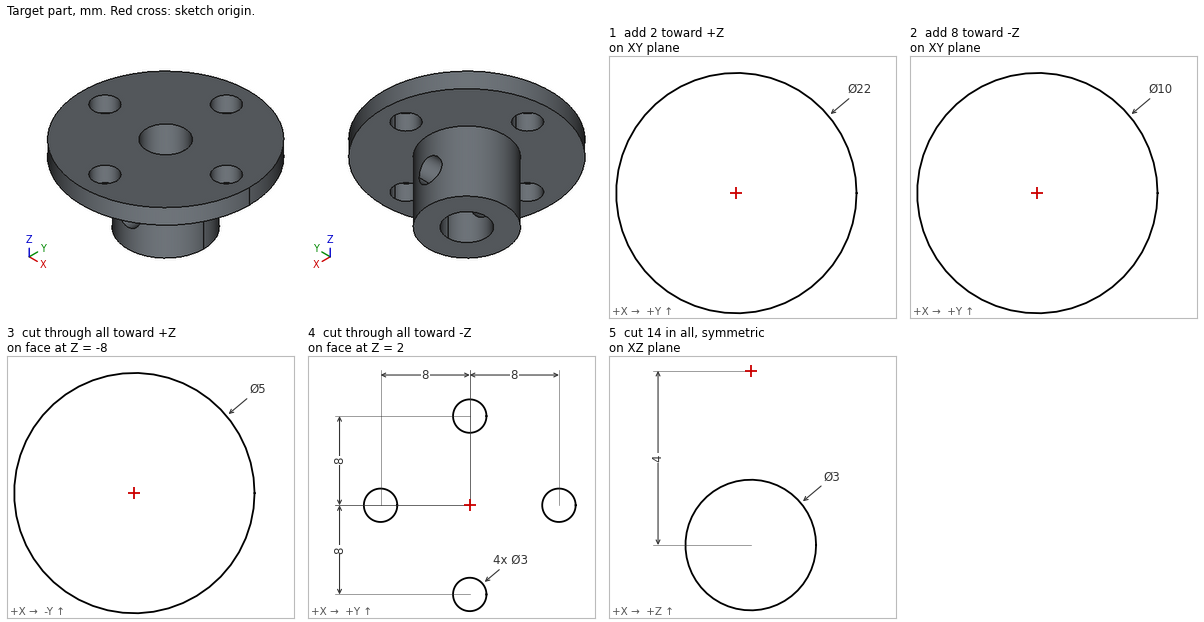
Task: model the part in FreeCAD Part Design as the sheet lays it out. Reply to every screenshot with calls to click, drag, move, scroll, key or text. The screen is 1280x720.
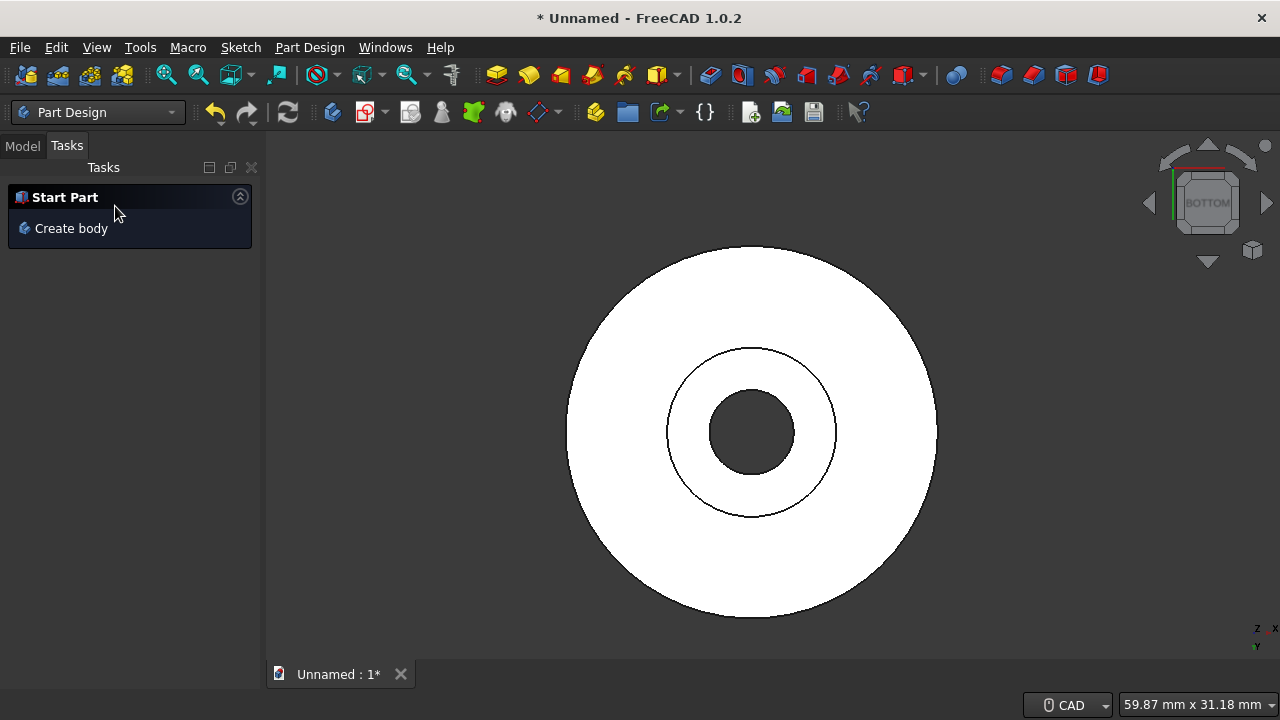
key(0)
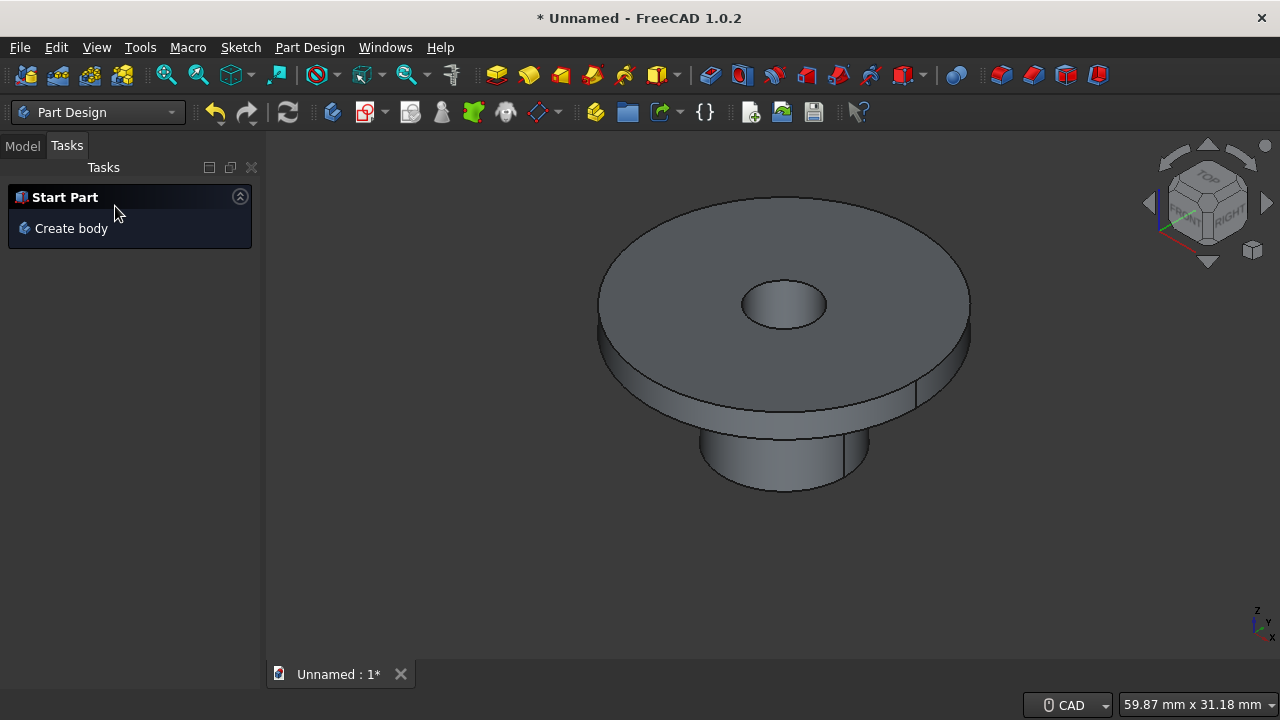
click(897, 282)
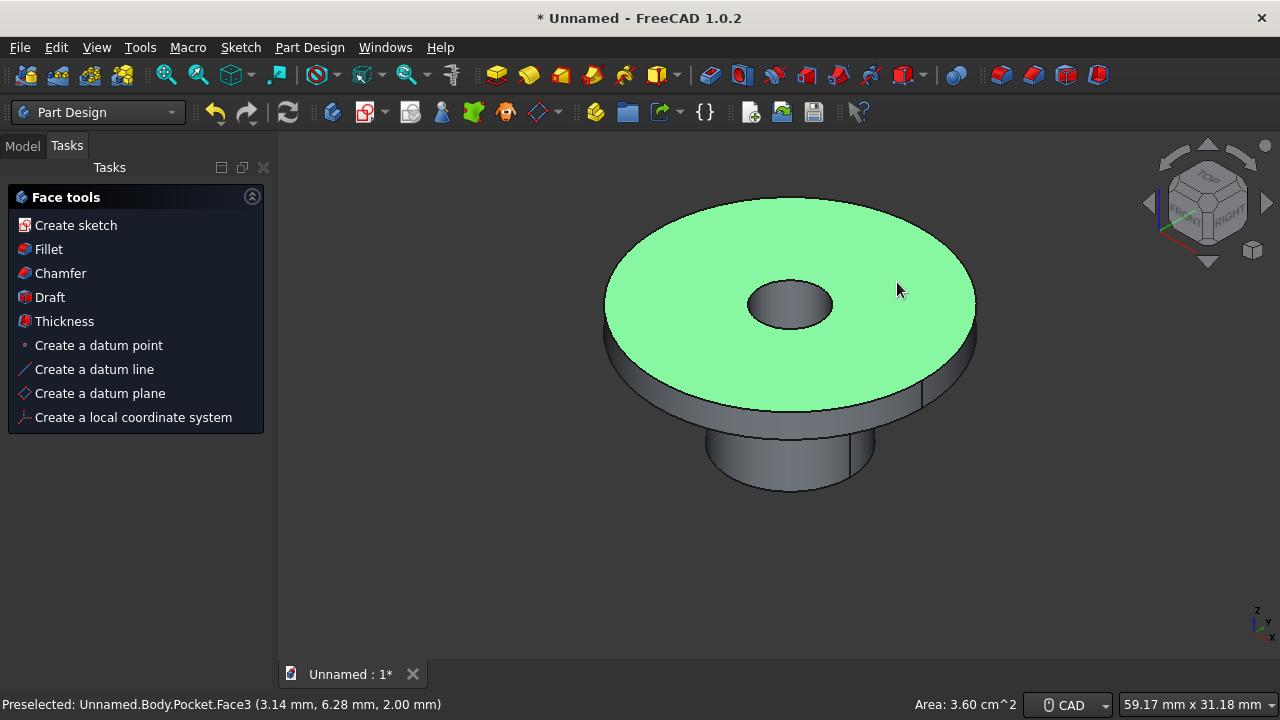
click(366, 112)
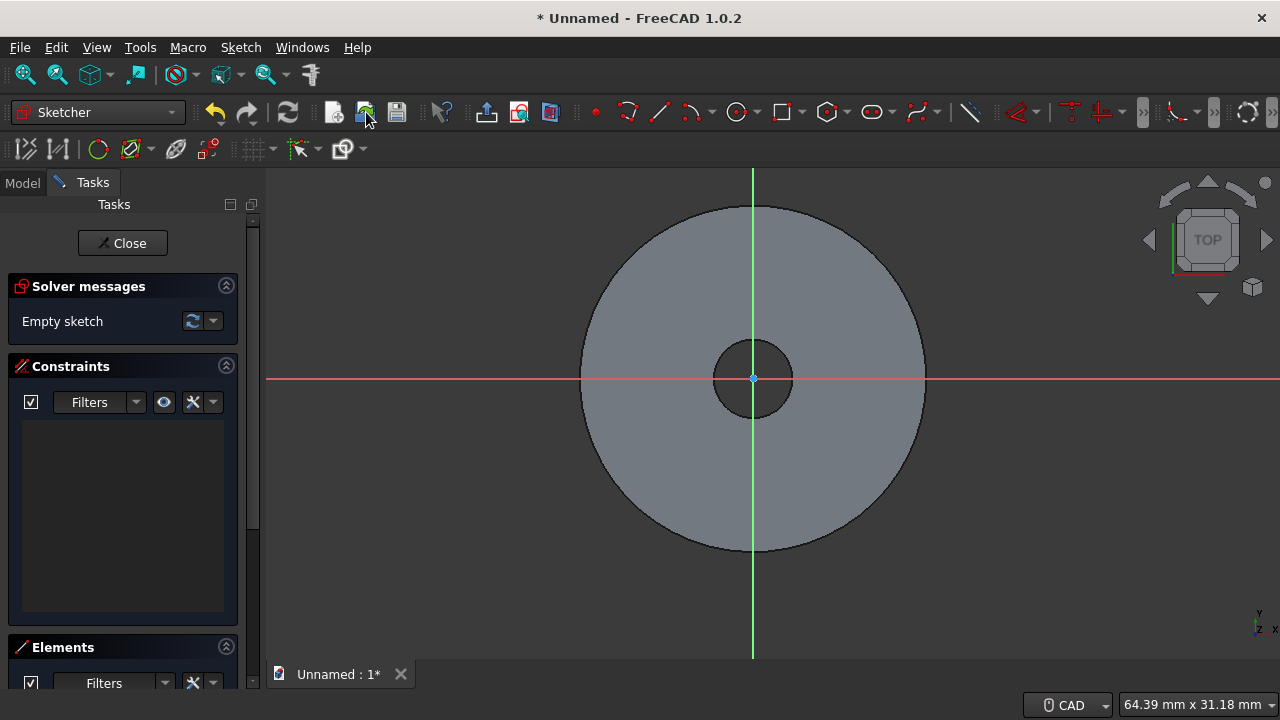
key(g)
key(c)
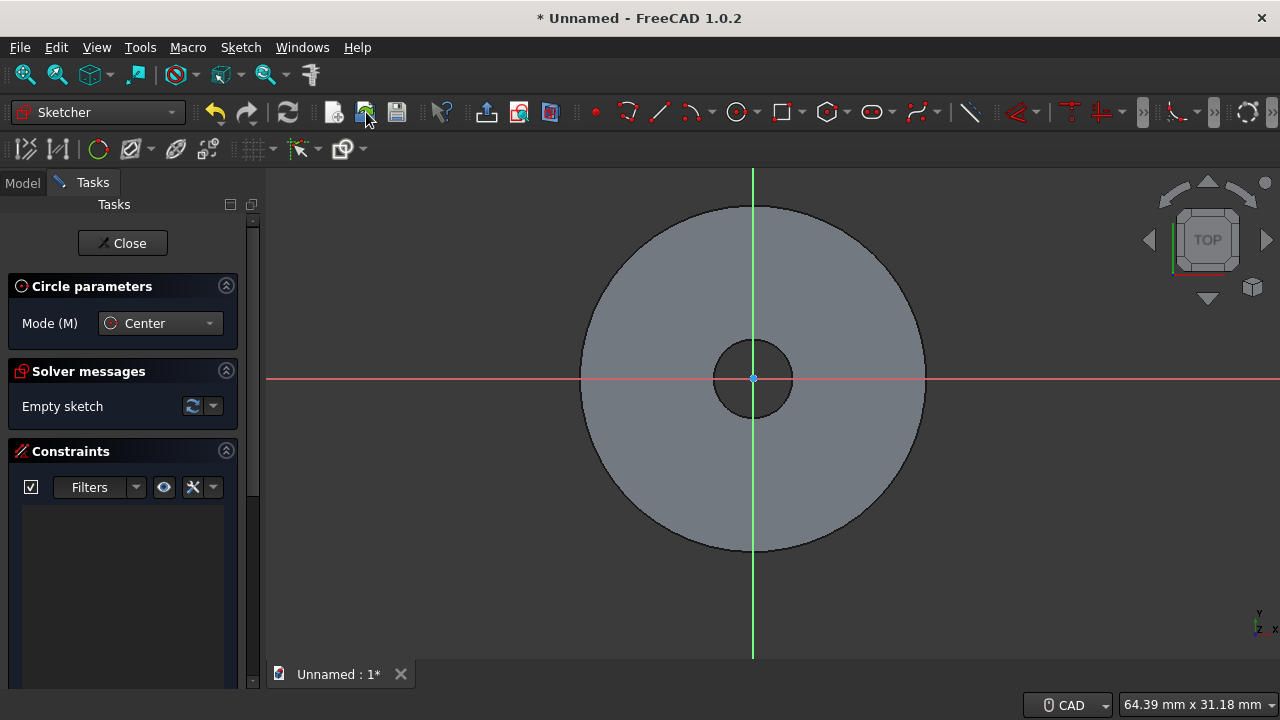
click(753, 505)
click(770, 488)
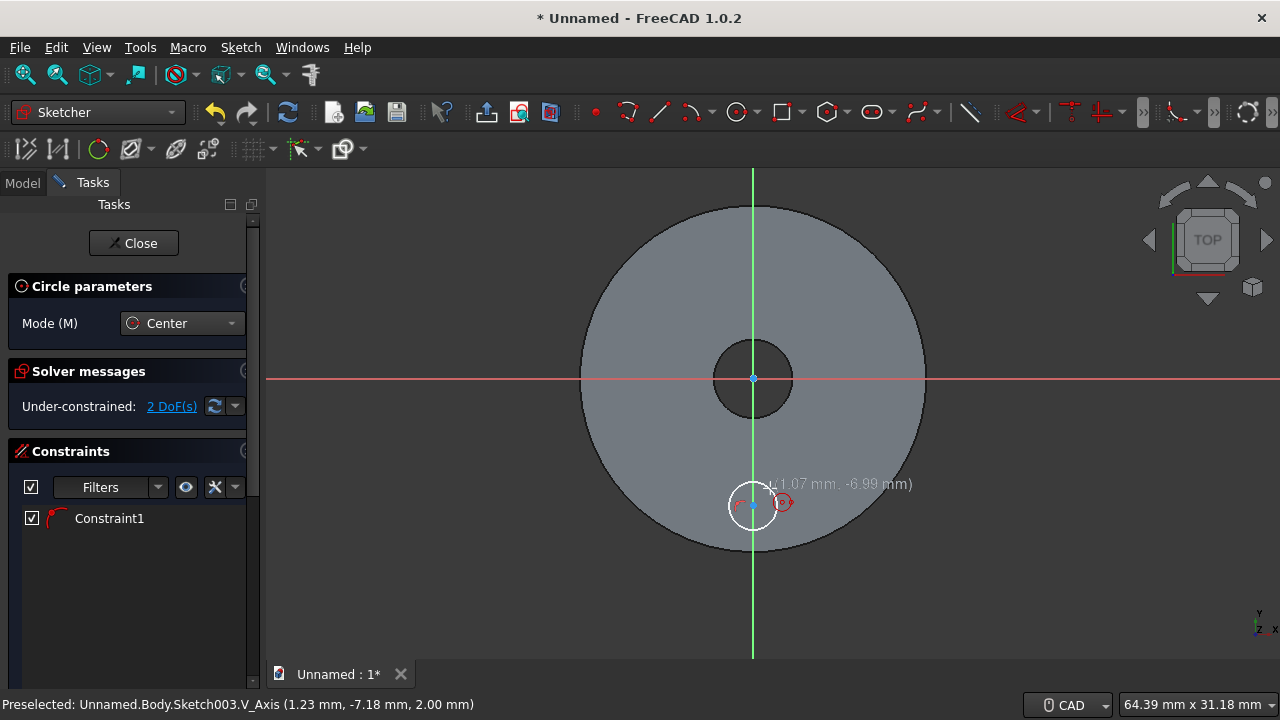
click(627, 379)
click(644, 362)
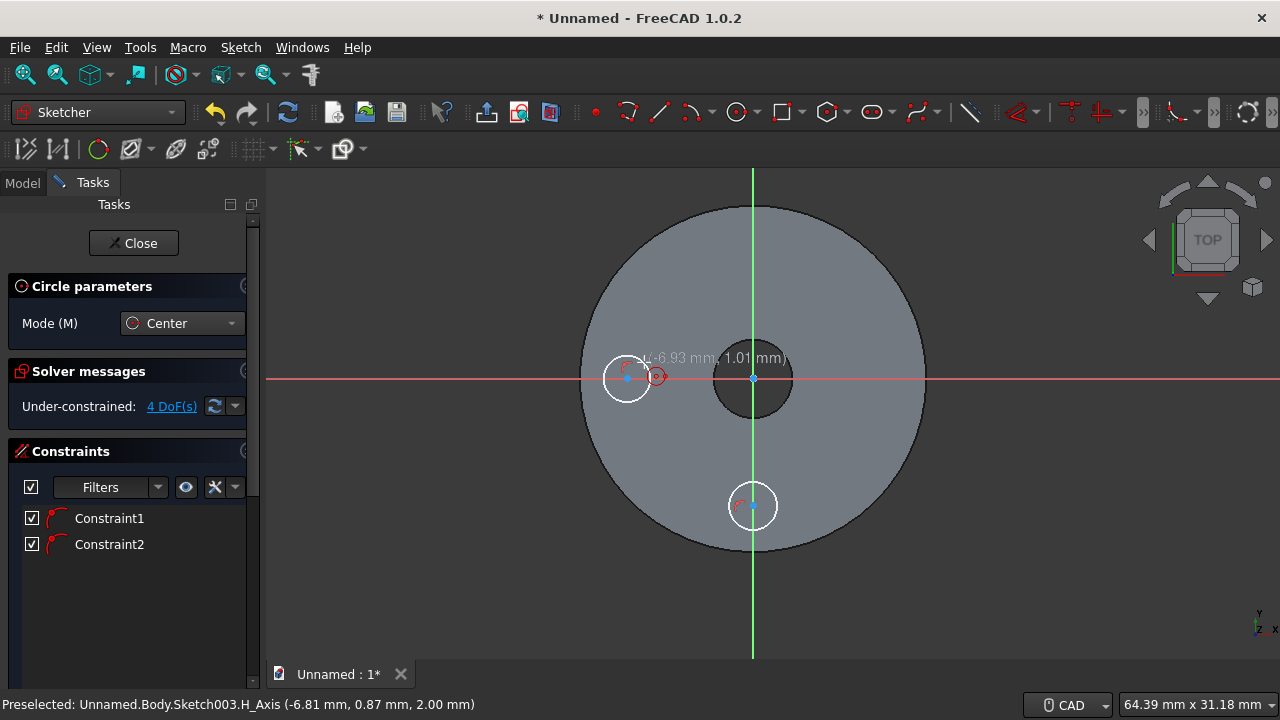
click(753, 253)
click(770, 236)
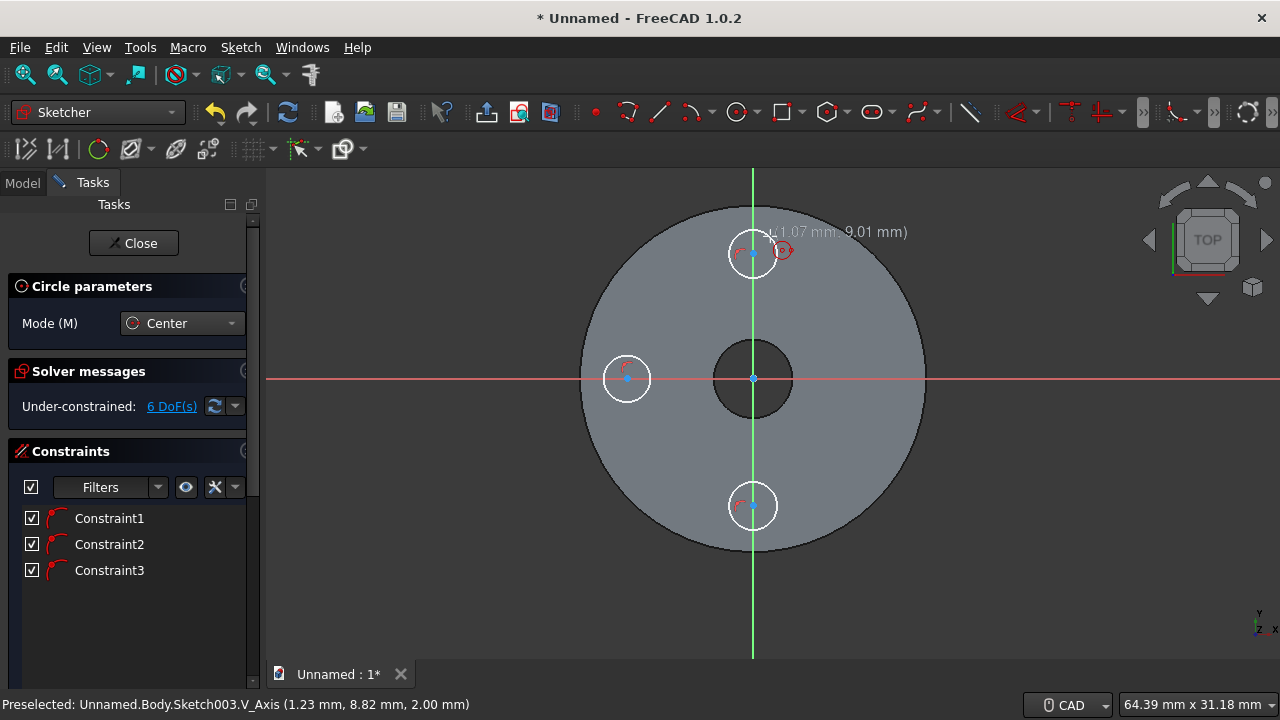
click(879, 379)
click(896, 362)
key(Escape)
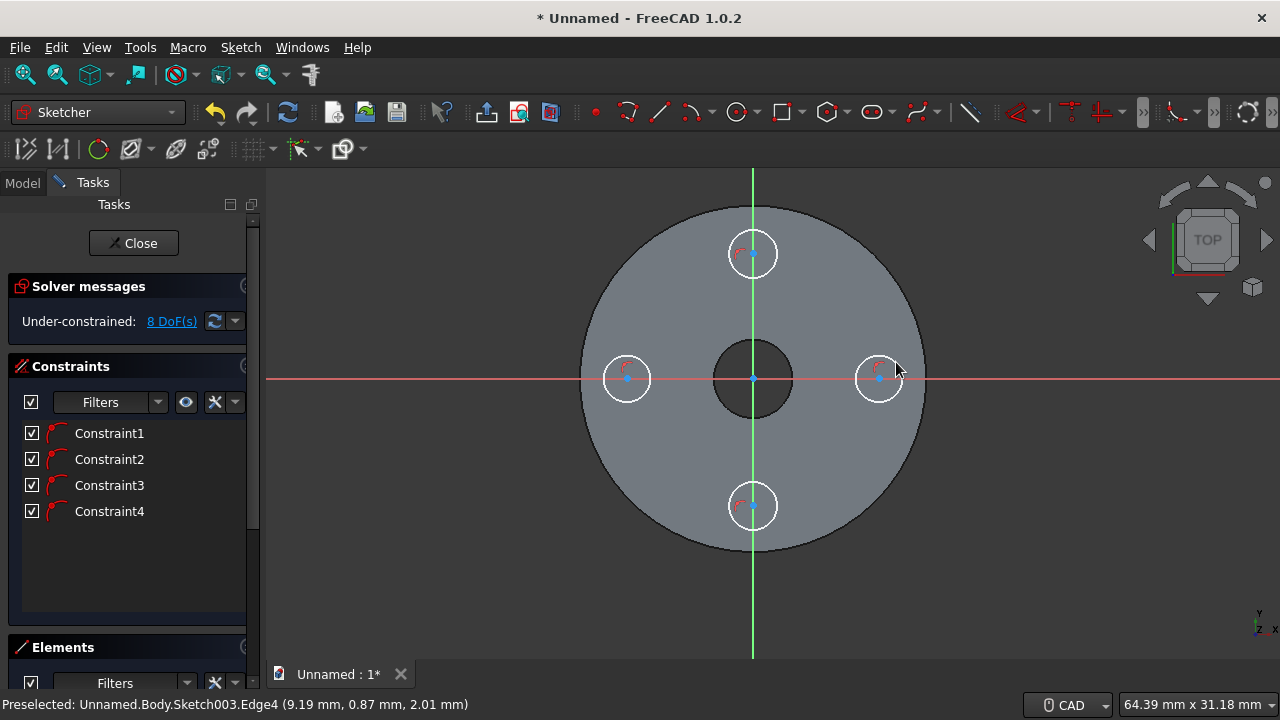
click(770, 489)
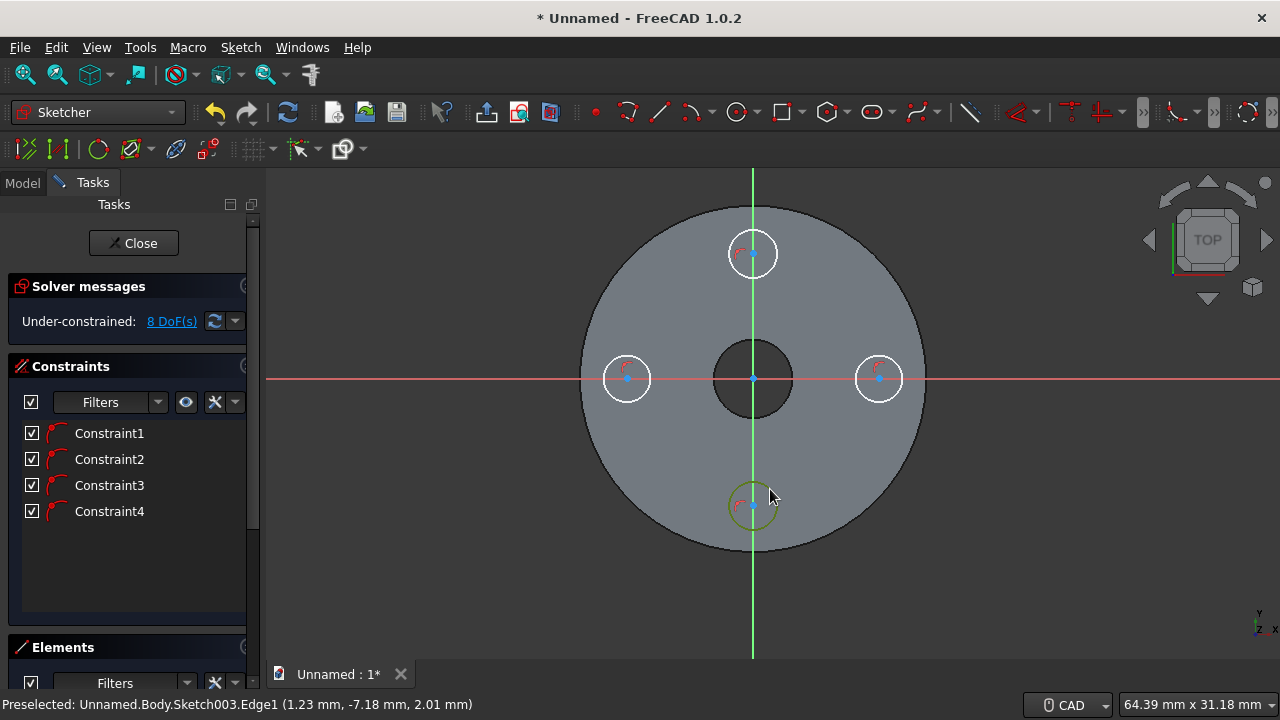
click(643, 362)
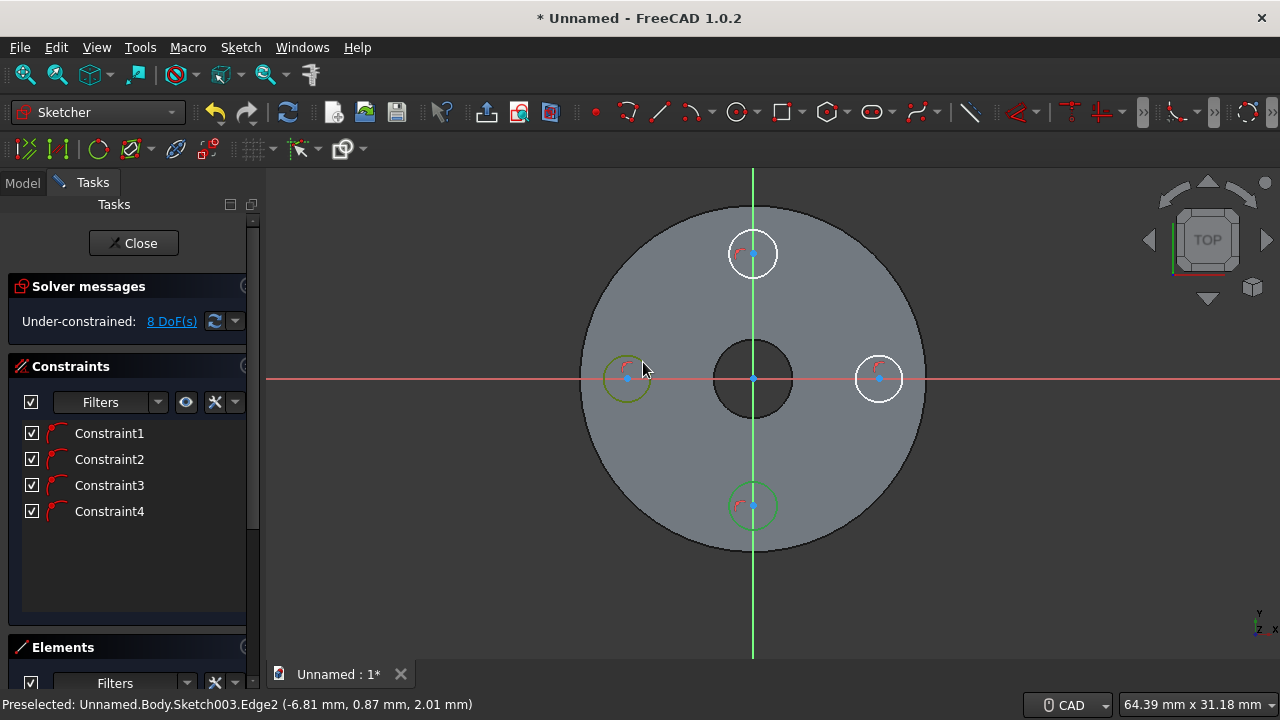
click(770, 237)